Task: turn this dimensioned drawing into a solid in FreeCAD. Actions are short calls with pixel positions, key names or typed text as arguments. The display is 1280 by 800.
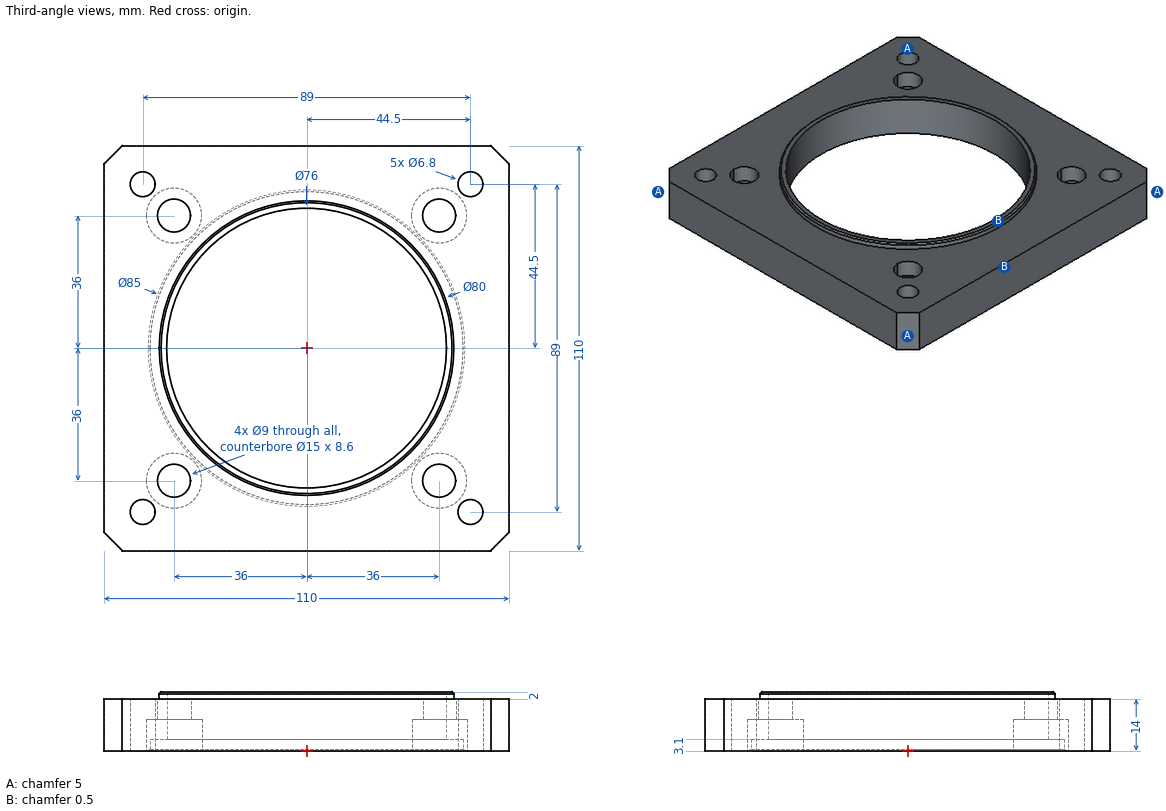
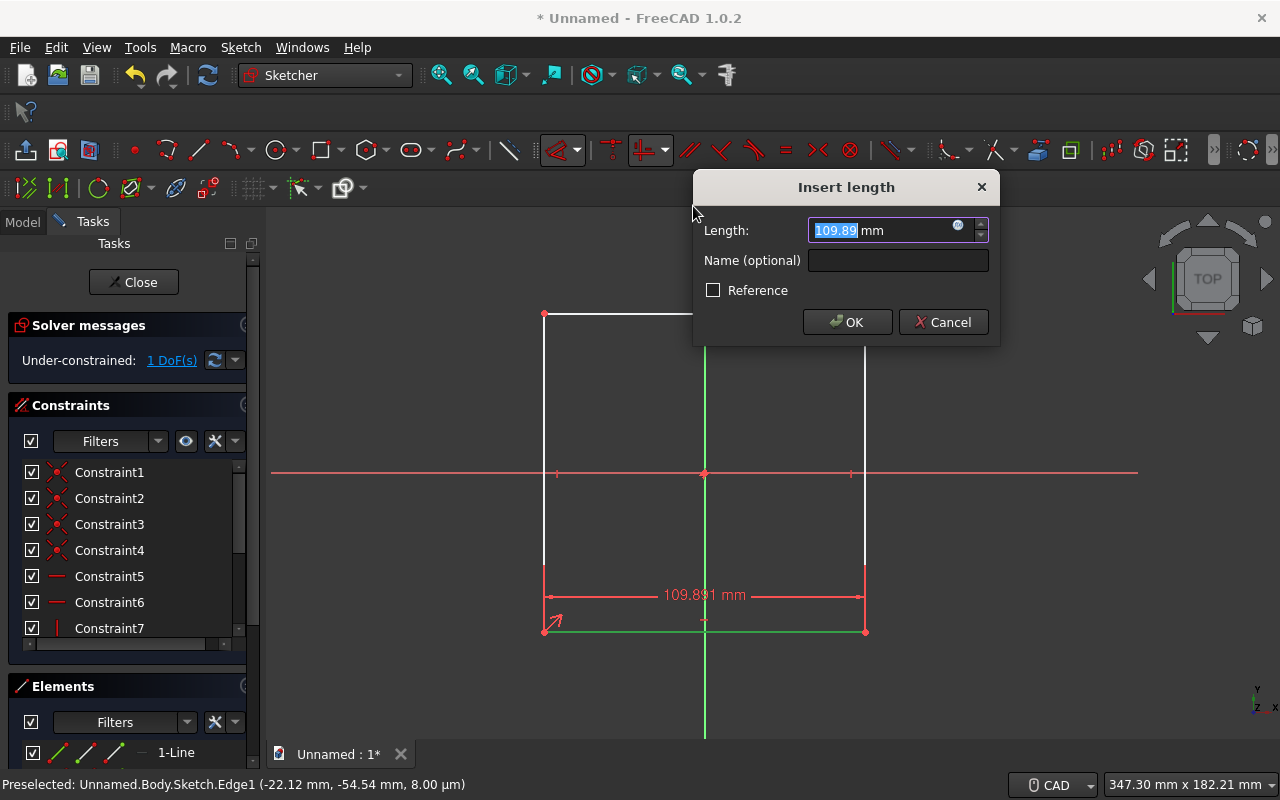
text(110)
key(Return)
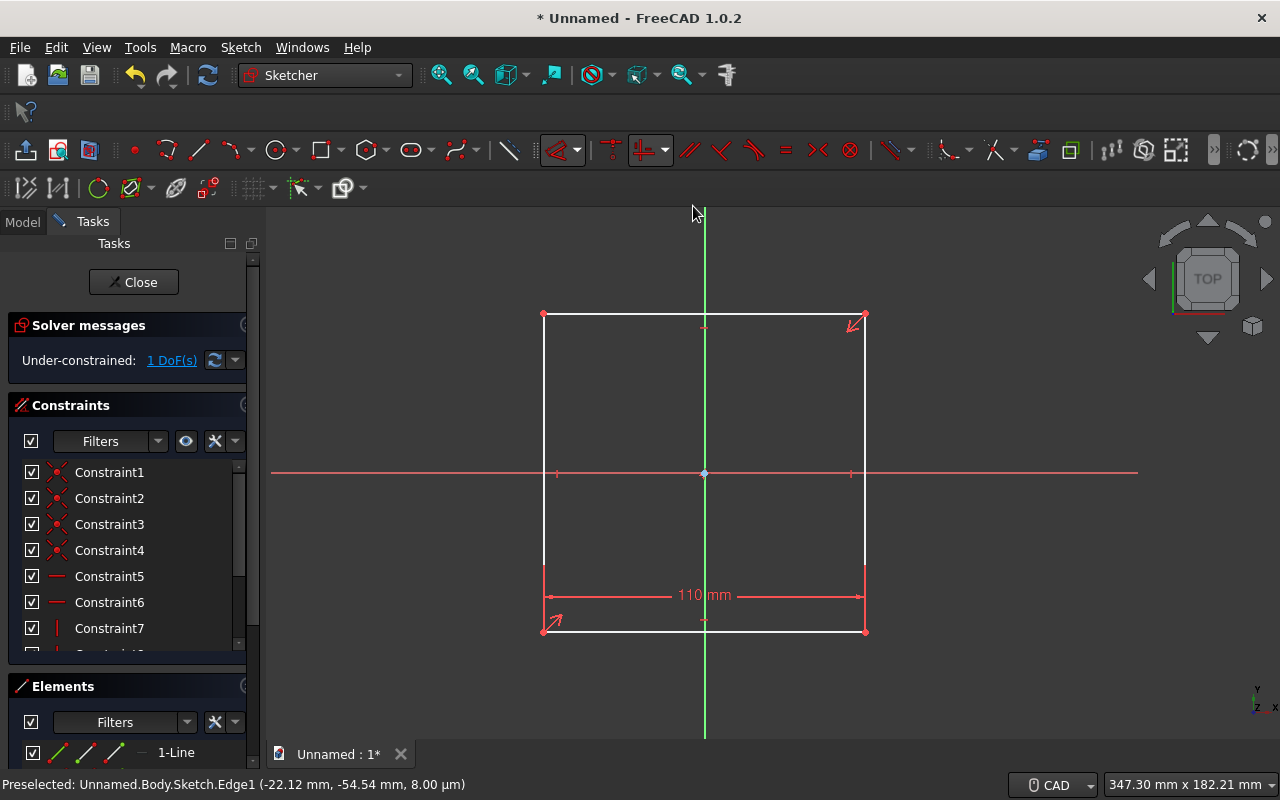
click(865, 537)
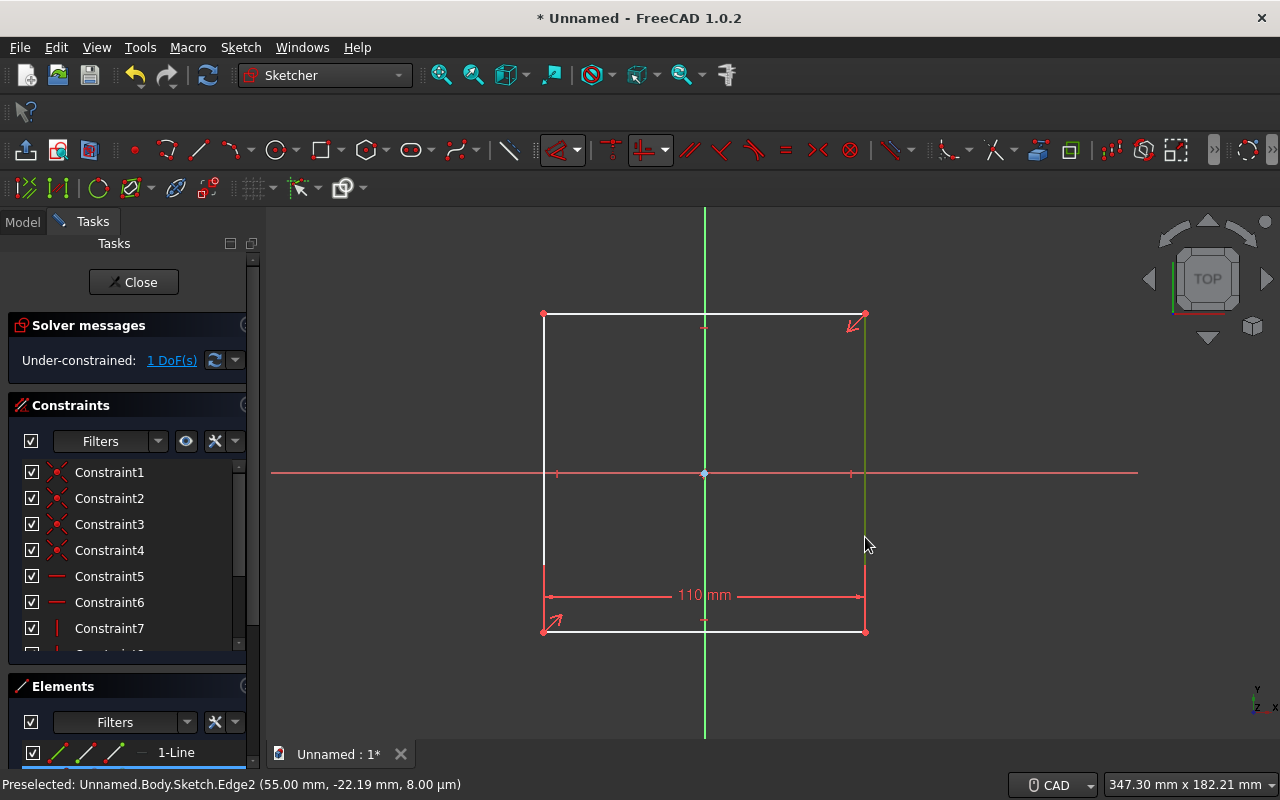
click(580, 150)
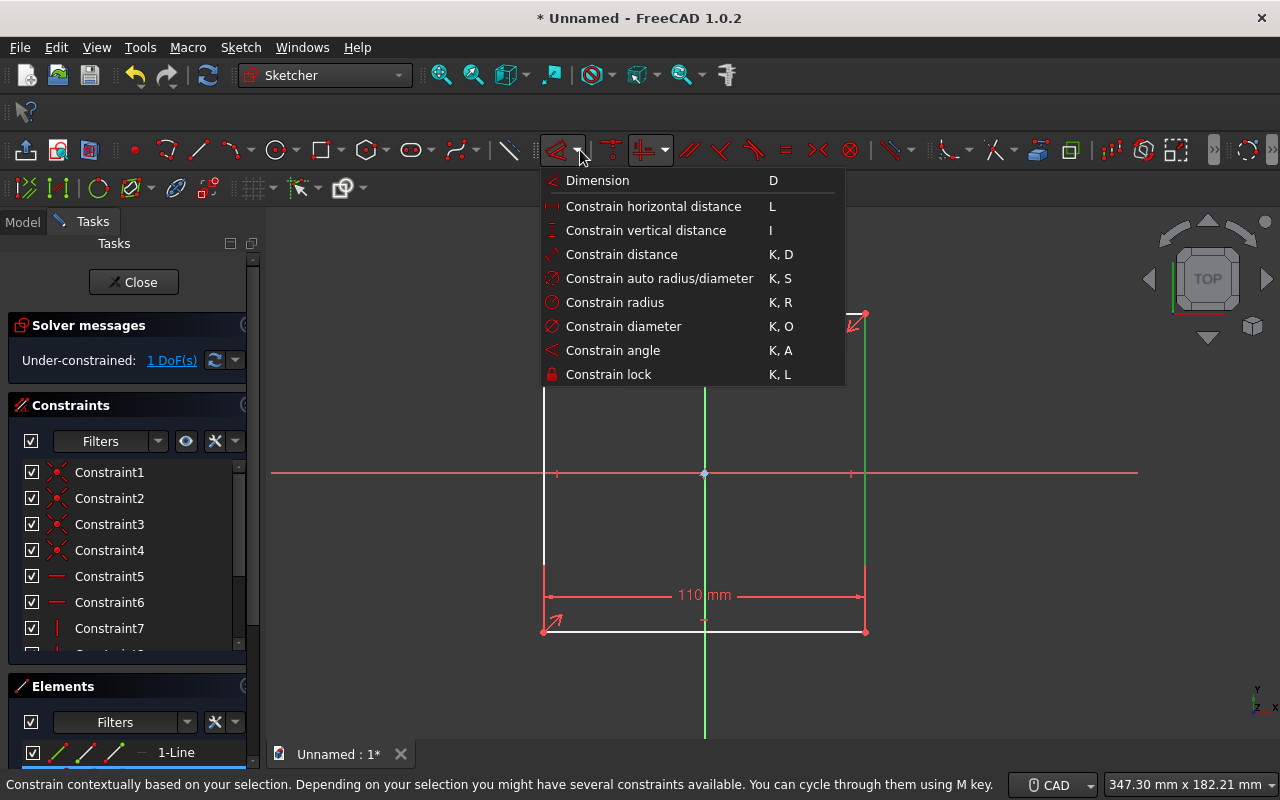
click(693, 230)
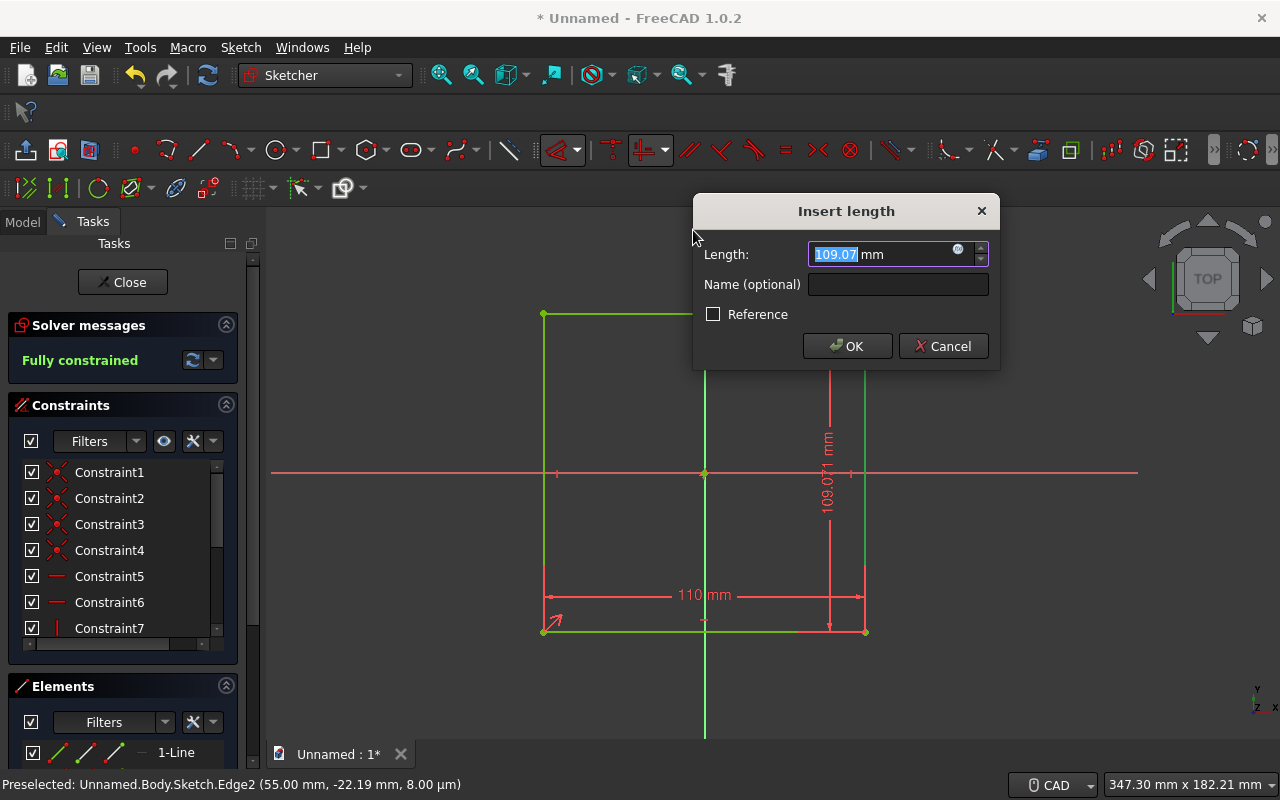
text(110)
key(Return)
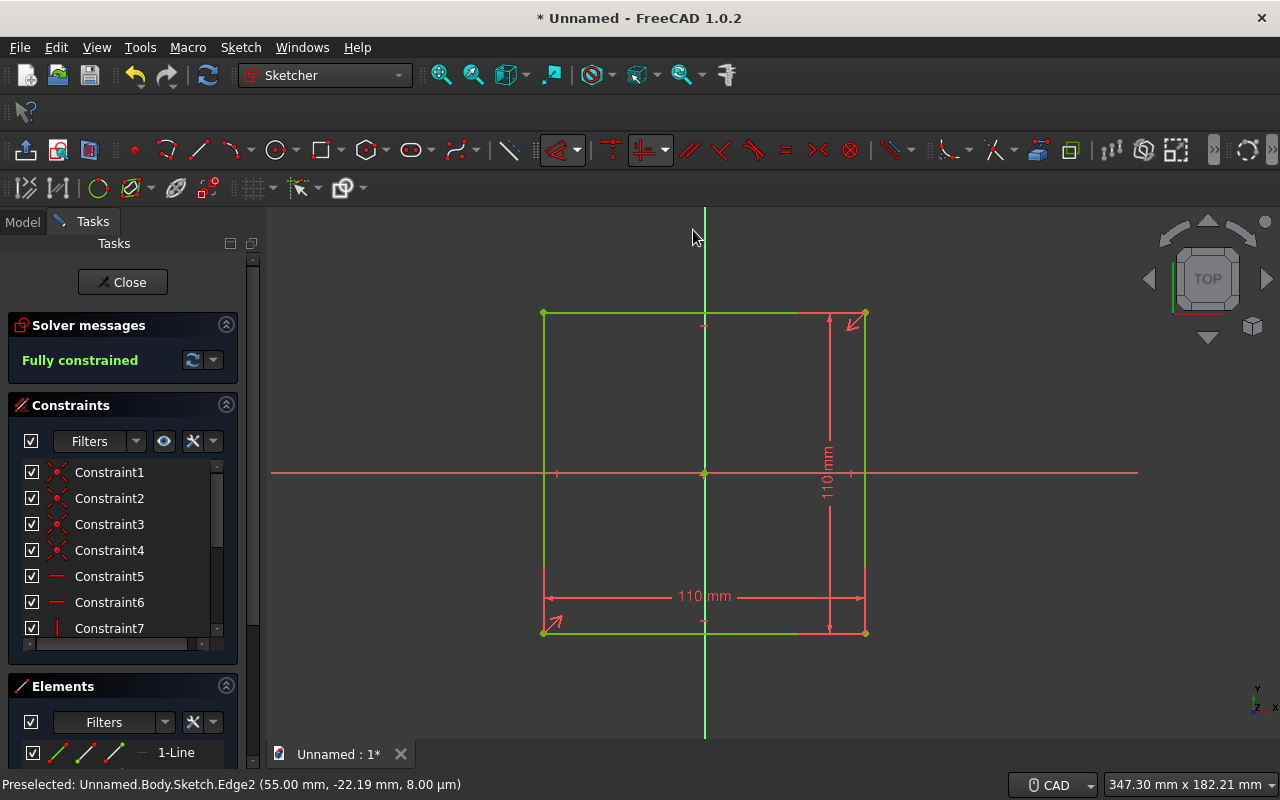
click(123, 282)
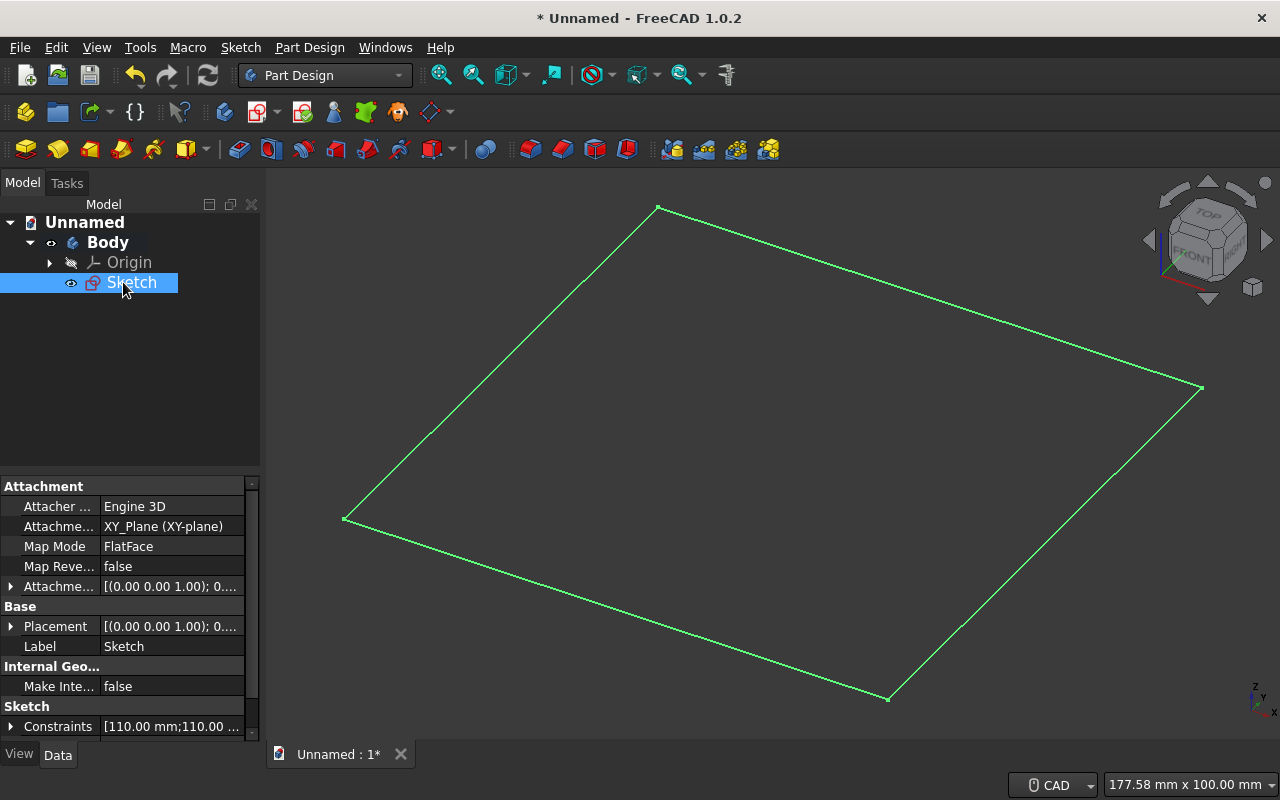
click(26, 150)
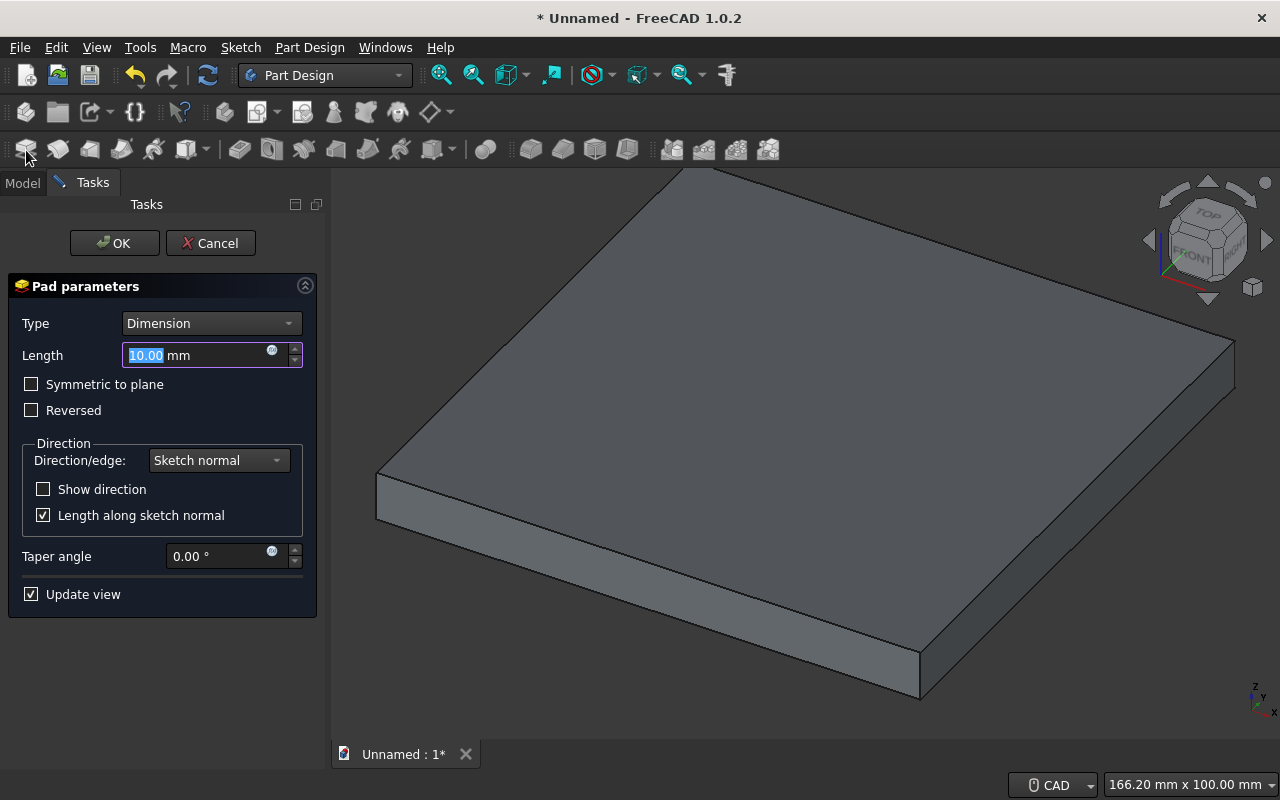
text(14)
key(Tab)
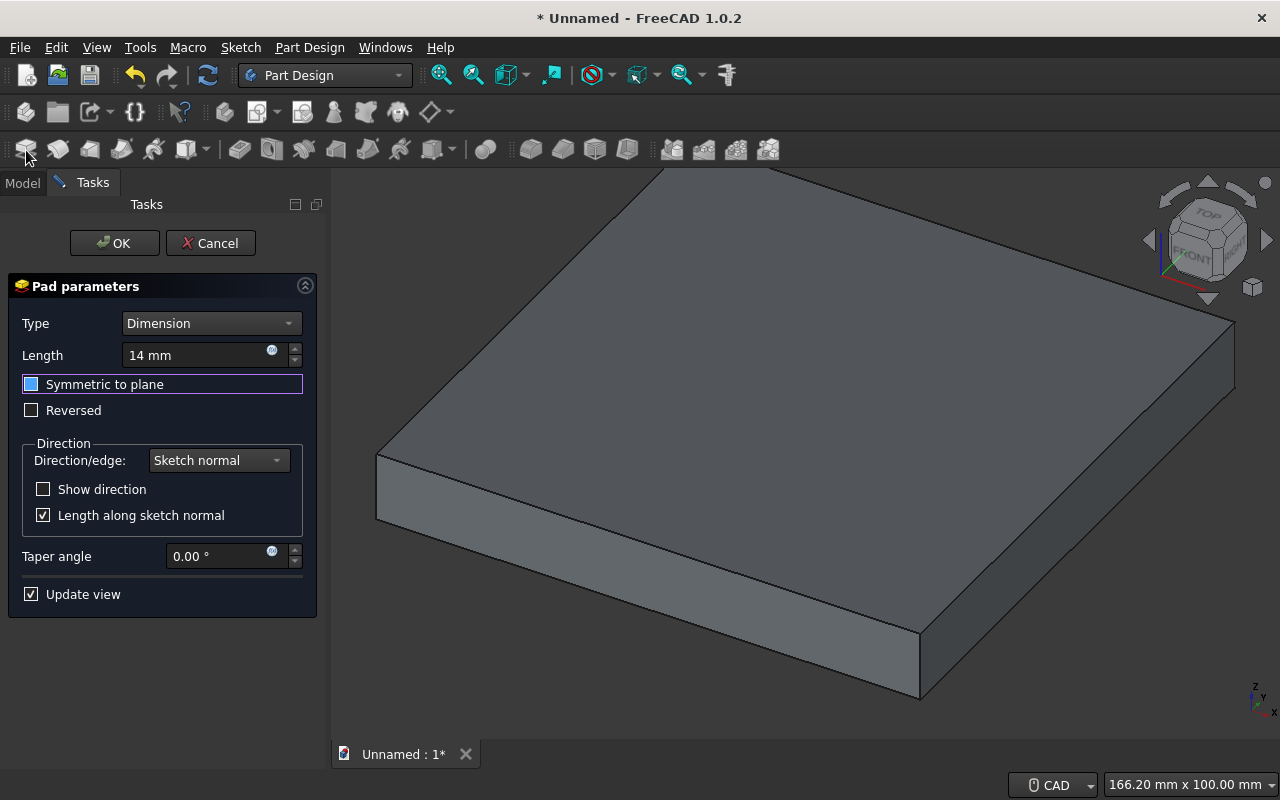
click(115, 243)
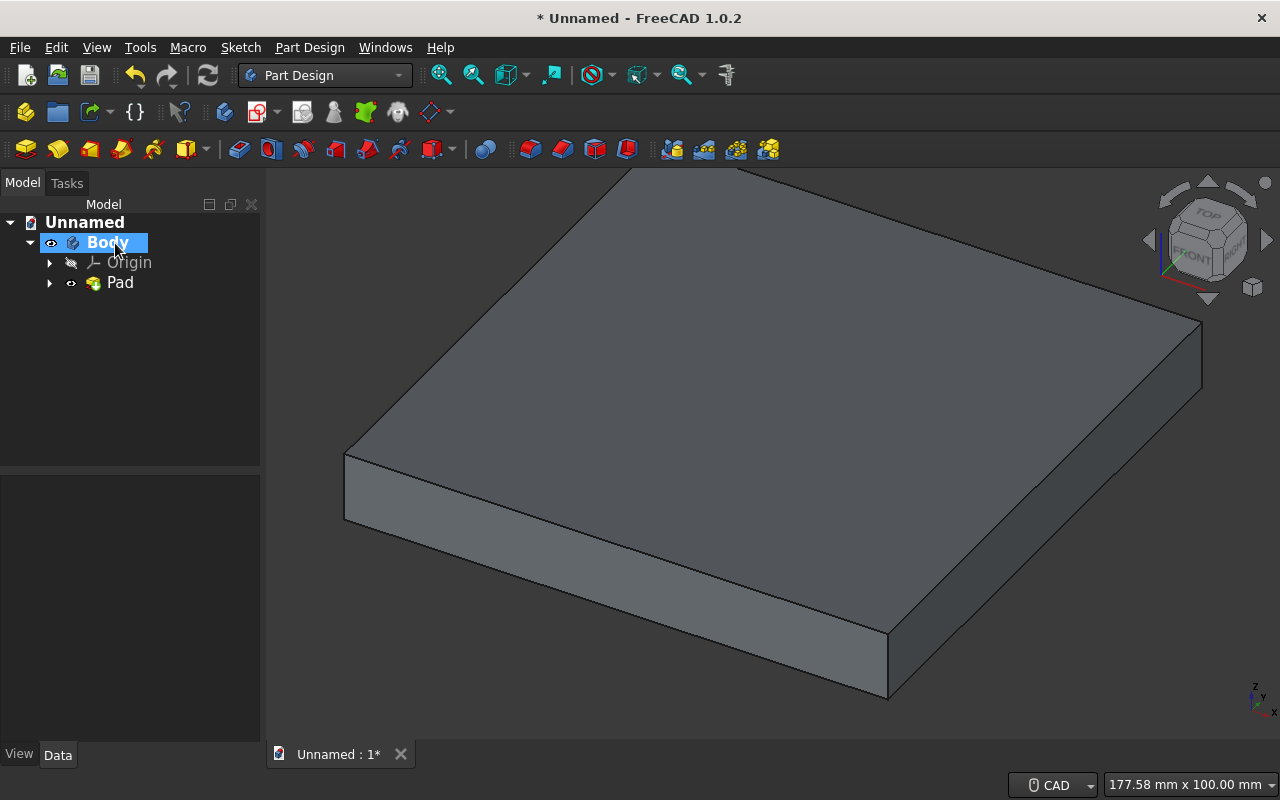
click(442, 76)